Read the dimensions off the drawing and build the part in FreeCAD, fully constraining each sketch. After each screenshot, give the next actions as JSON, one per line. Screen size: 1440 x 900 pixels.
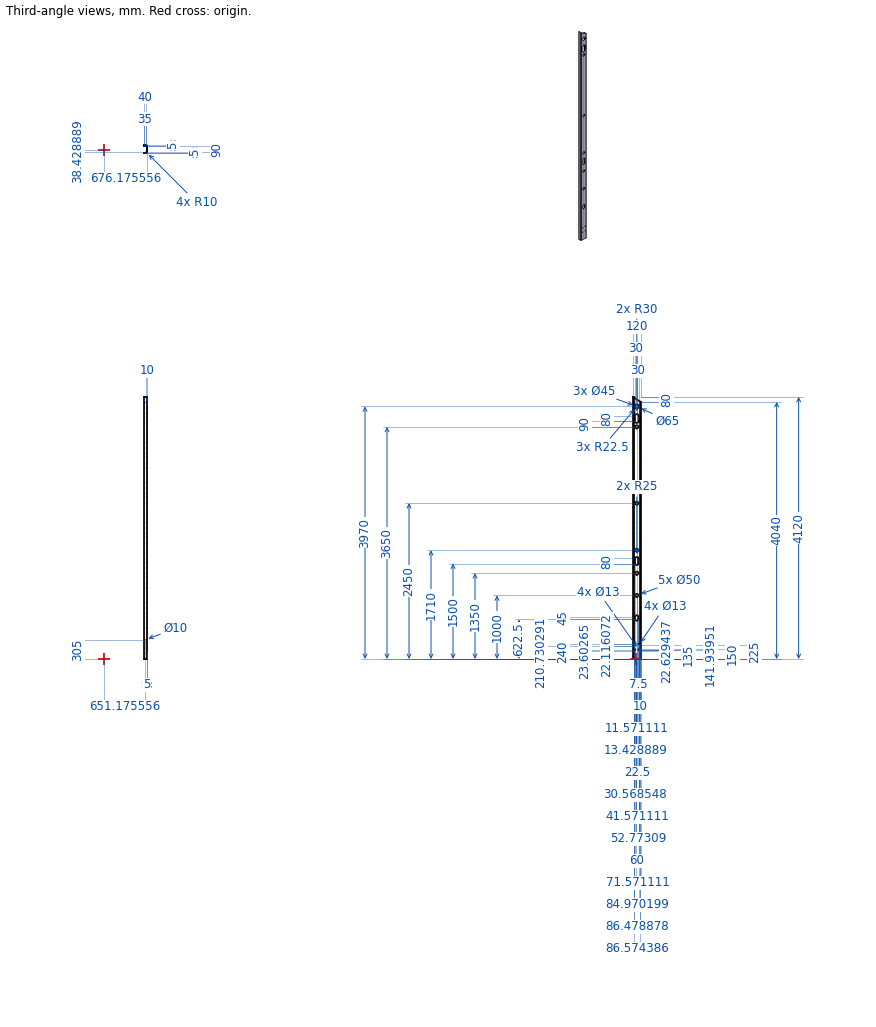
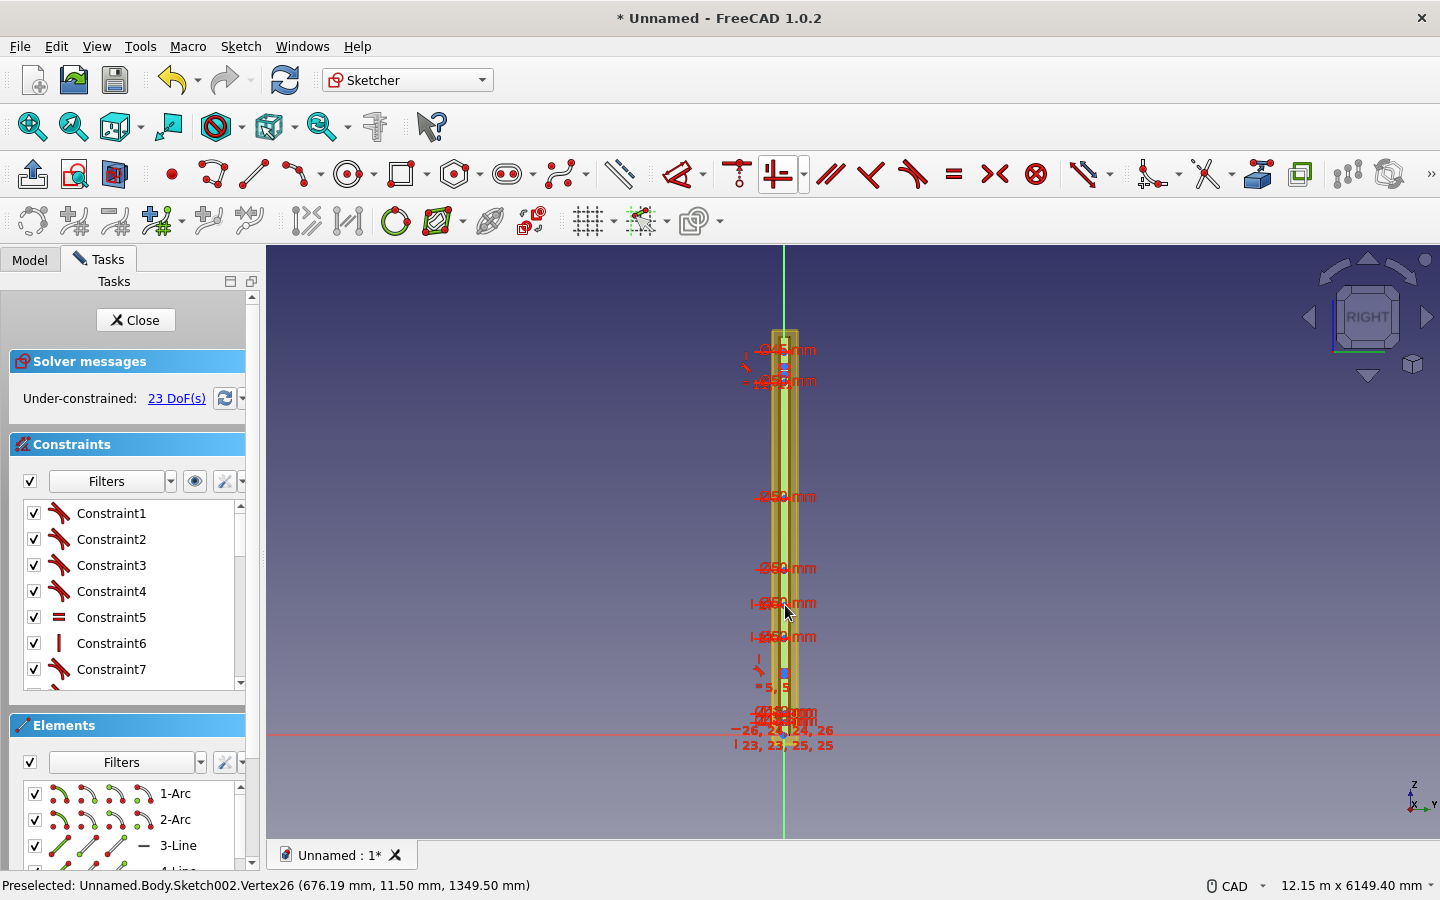
{"action": "left_click", "coordinate": [785, 605]}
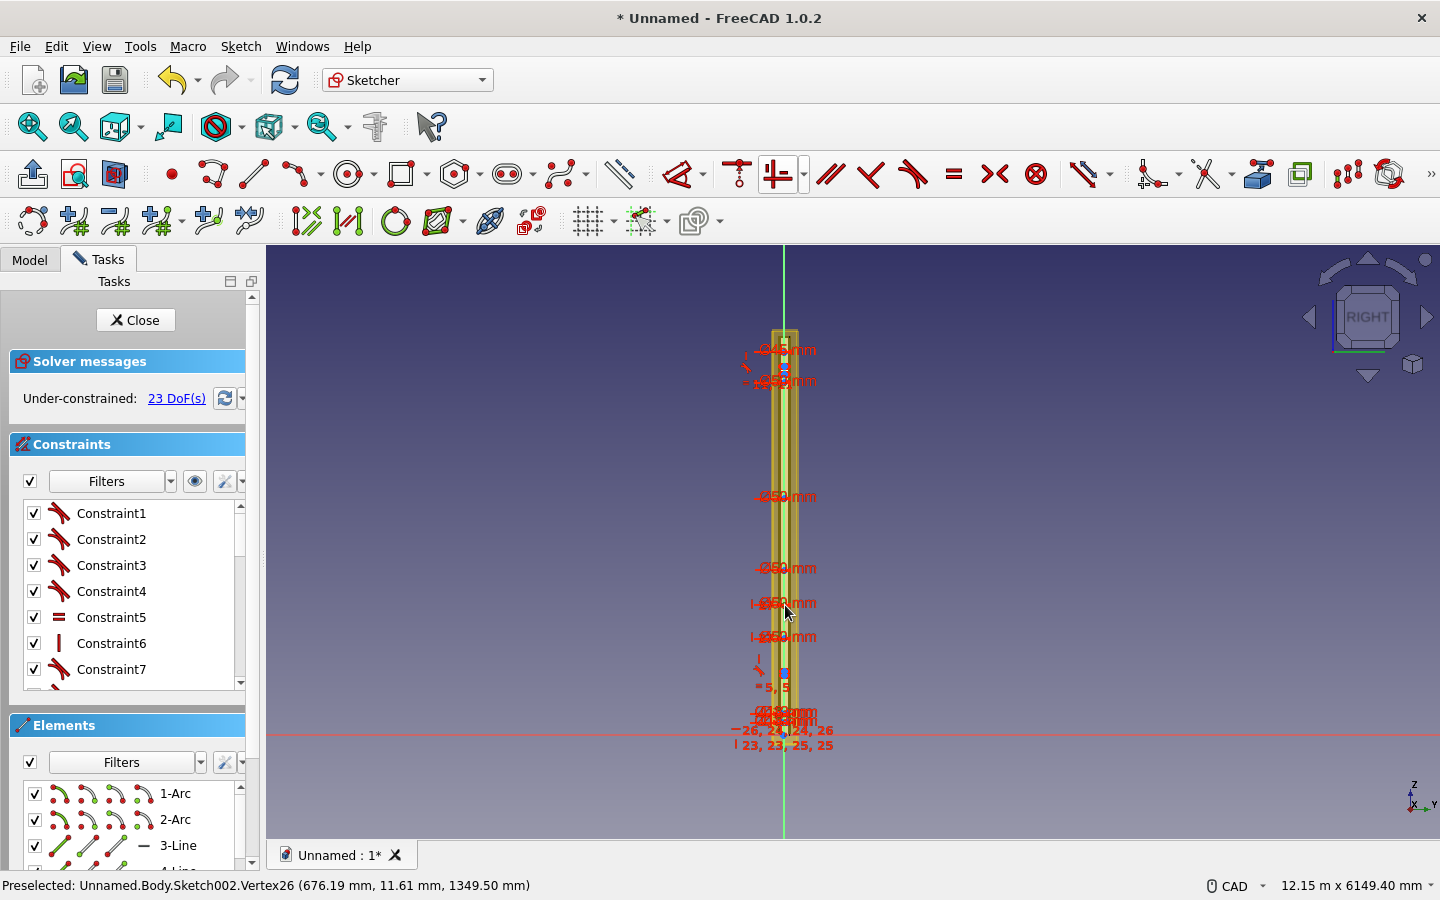
{"action": "left_click", "coordinate": [785, 570]}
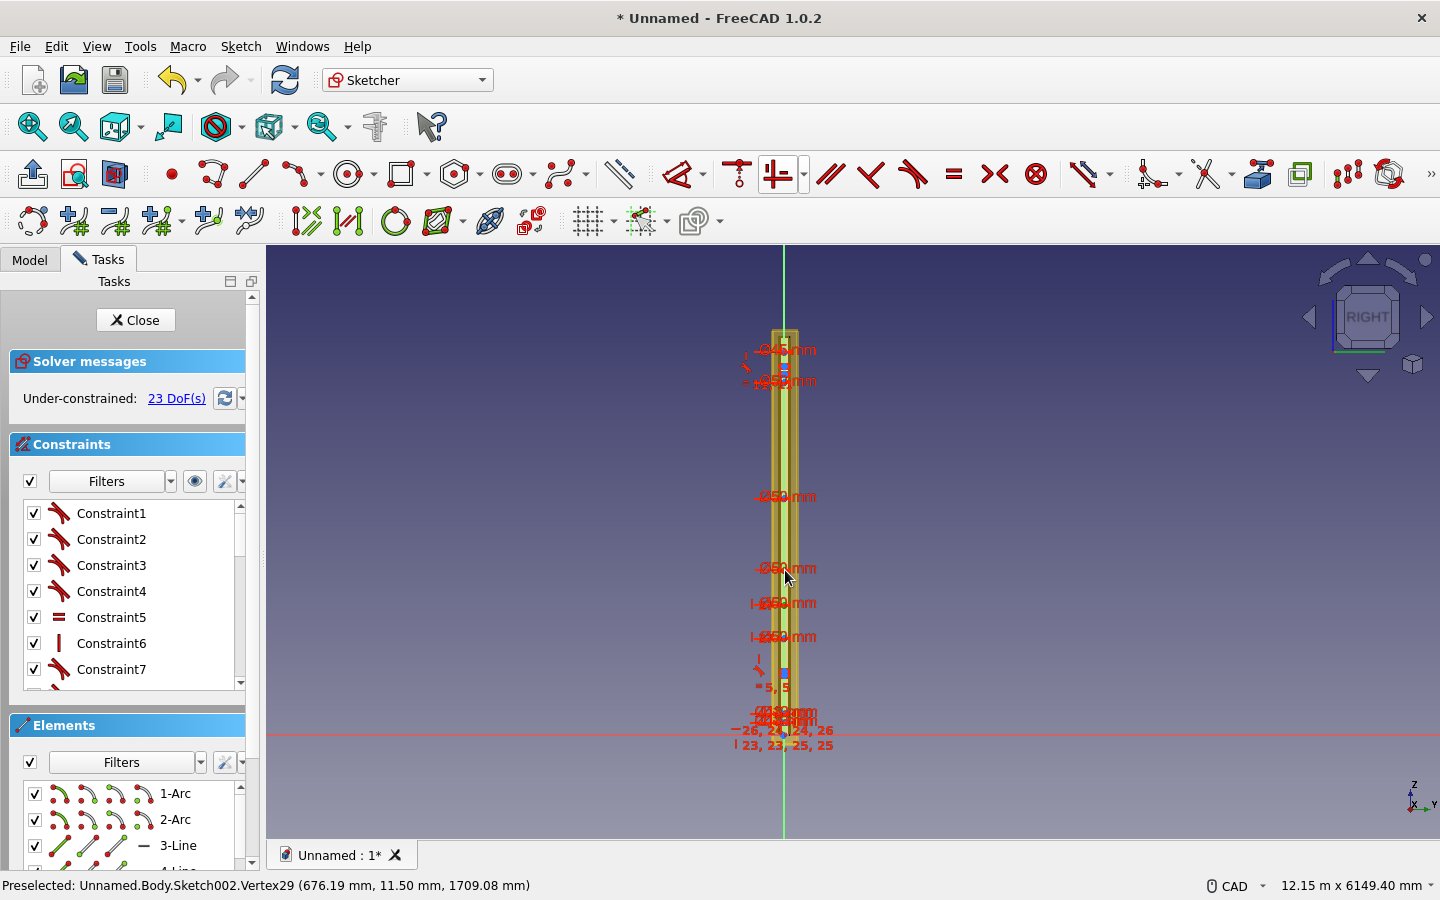
{"action": "key", "text": "v"}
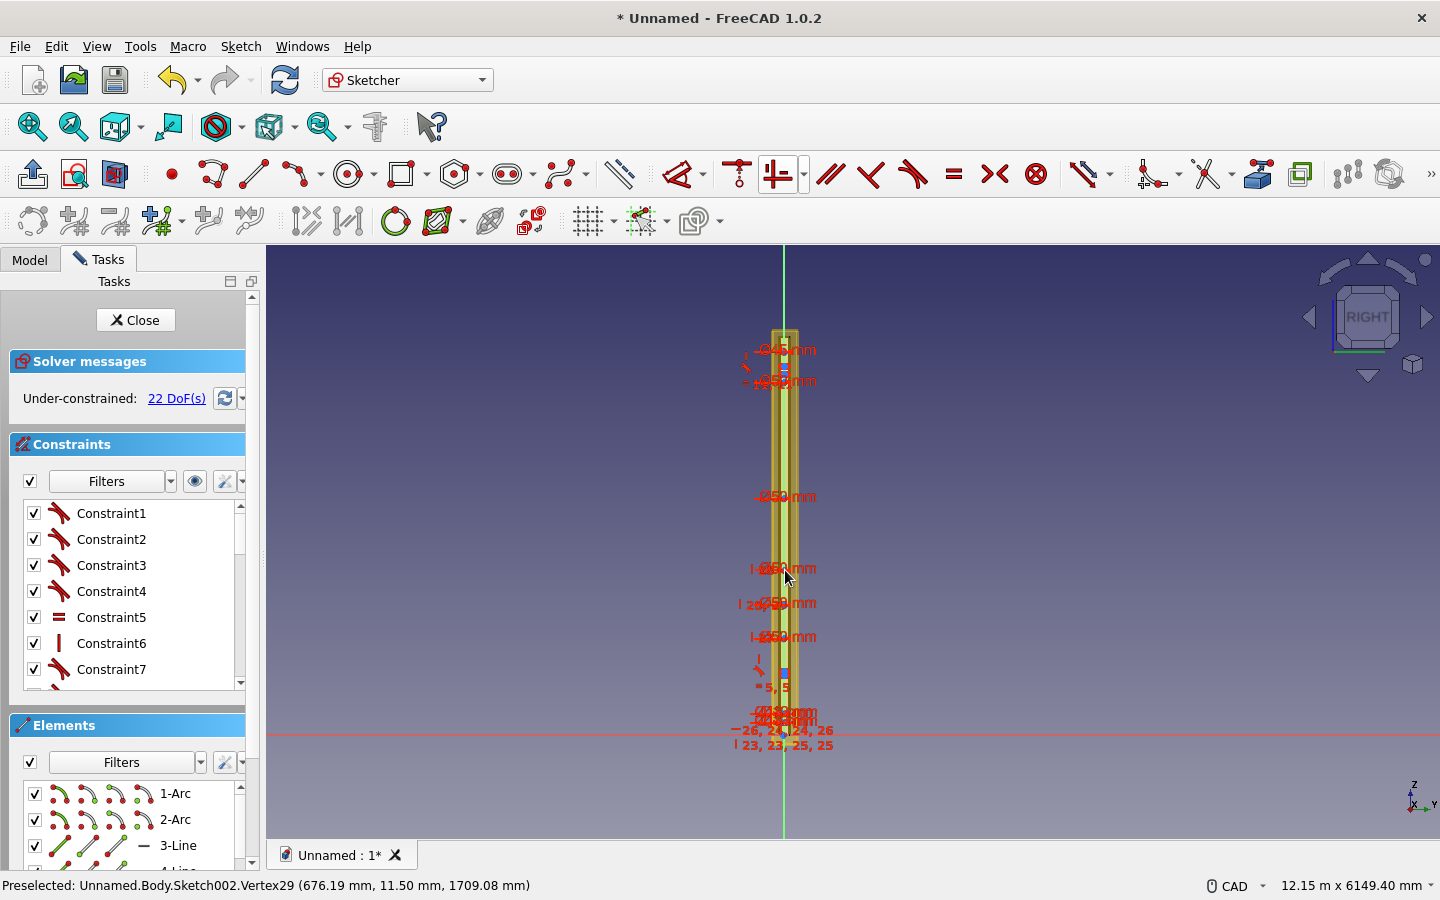
{"action": "left_click", "coordinate": [785, 570]}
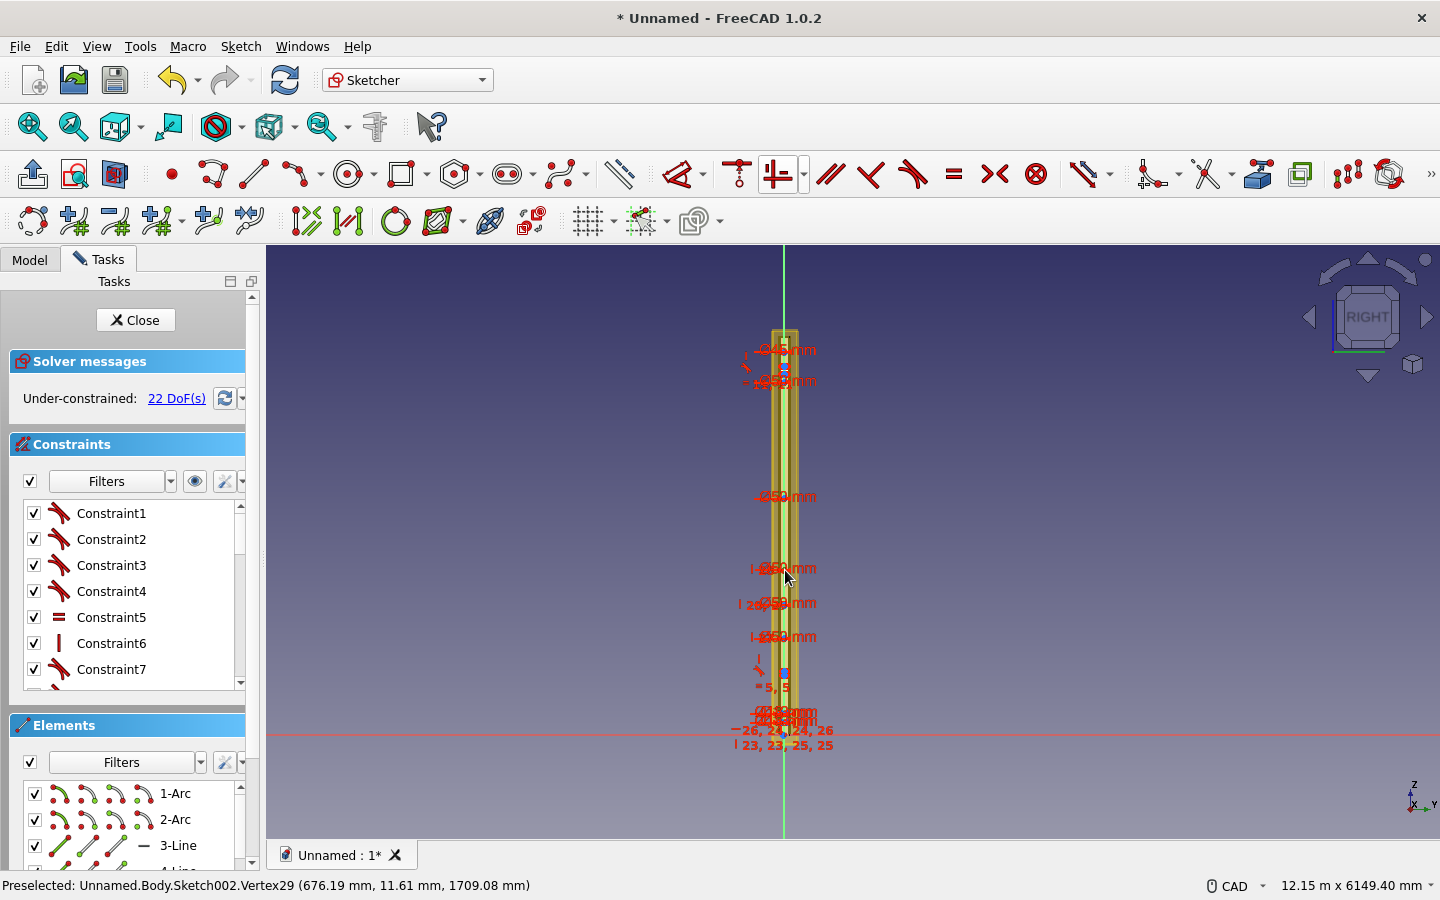
{"action": "left_click", "coordinate": [785, 499]}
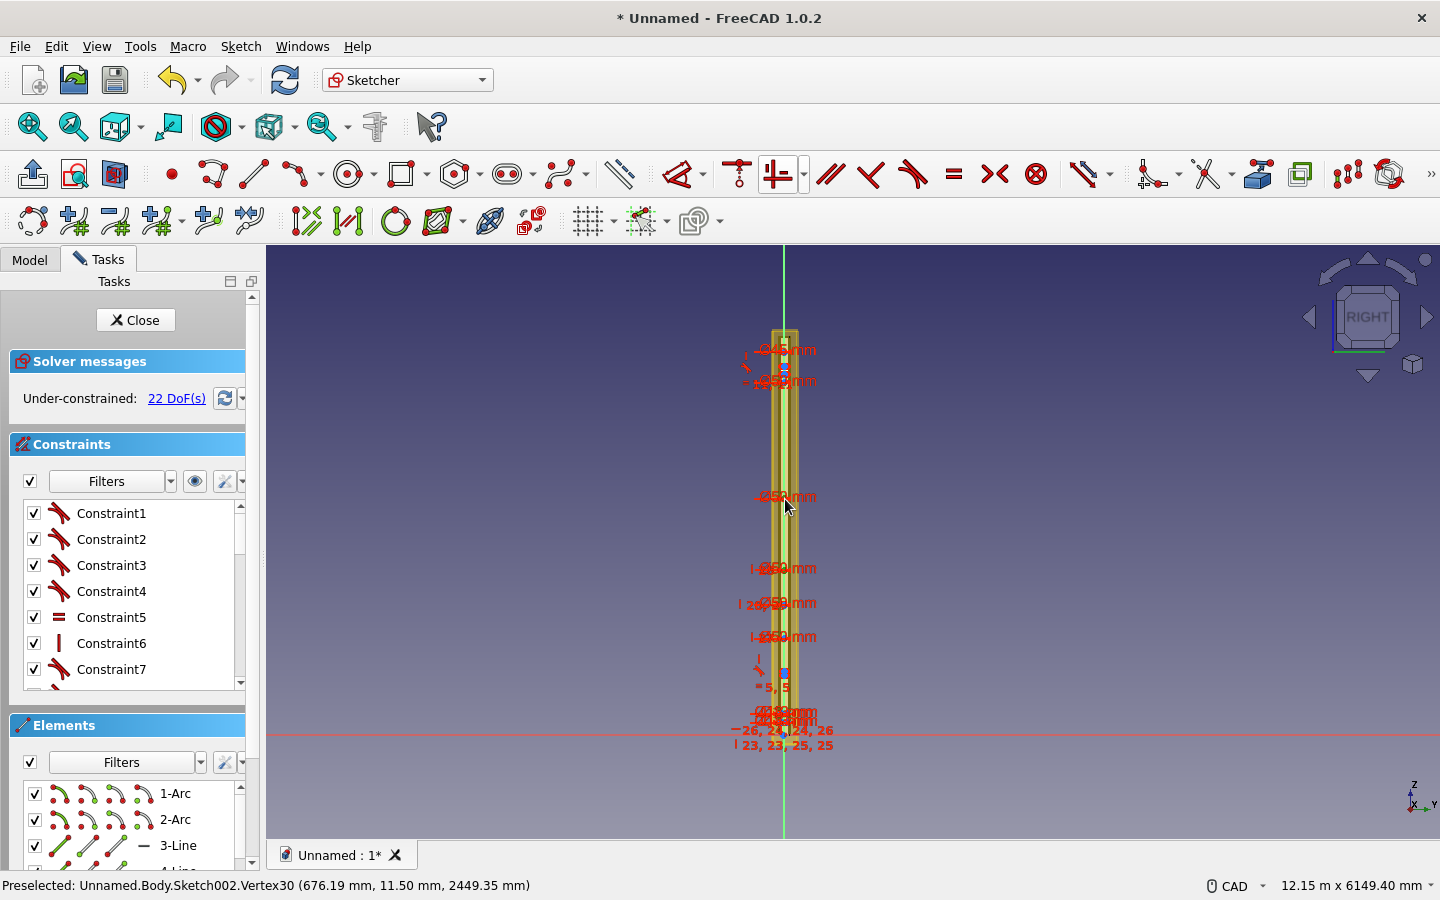
{"action": "key", "text": "v"}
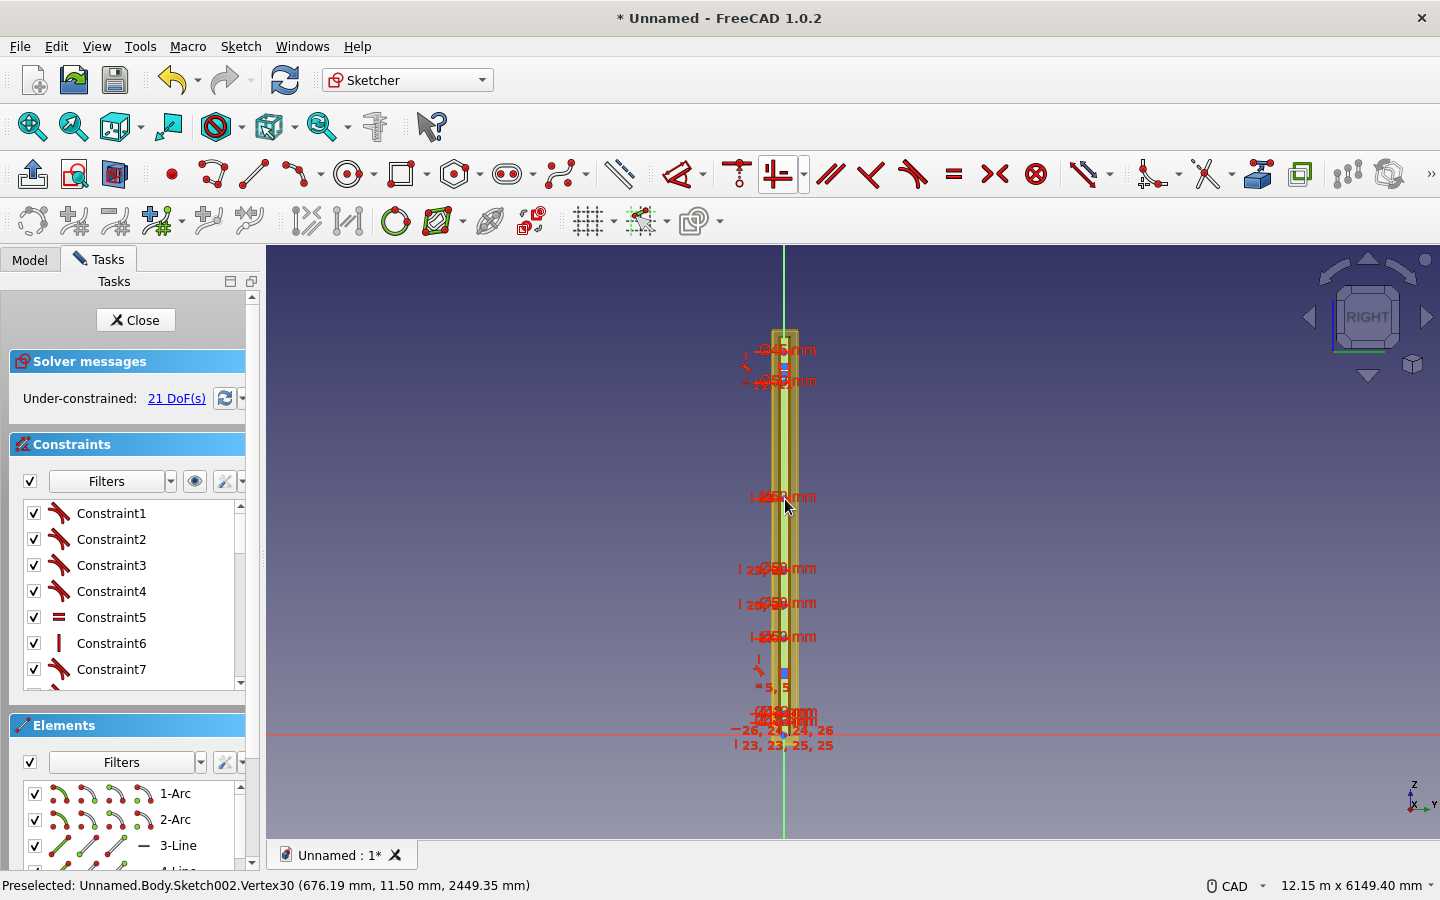
{"action": "scroll", "coordinate": [785, 383], "scroll_direction": "up", "scroll_amount": 2}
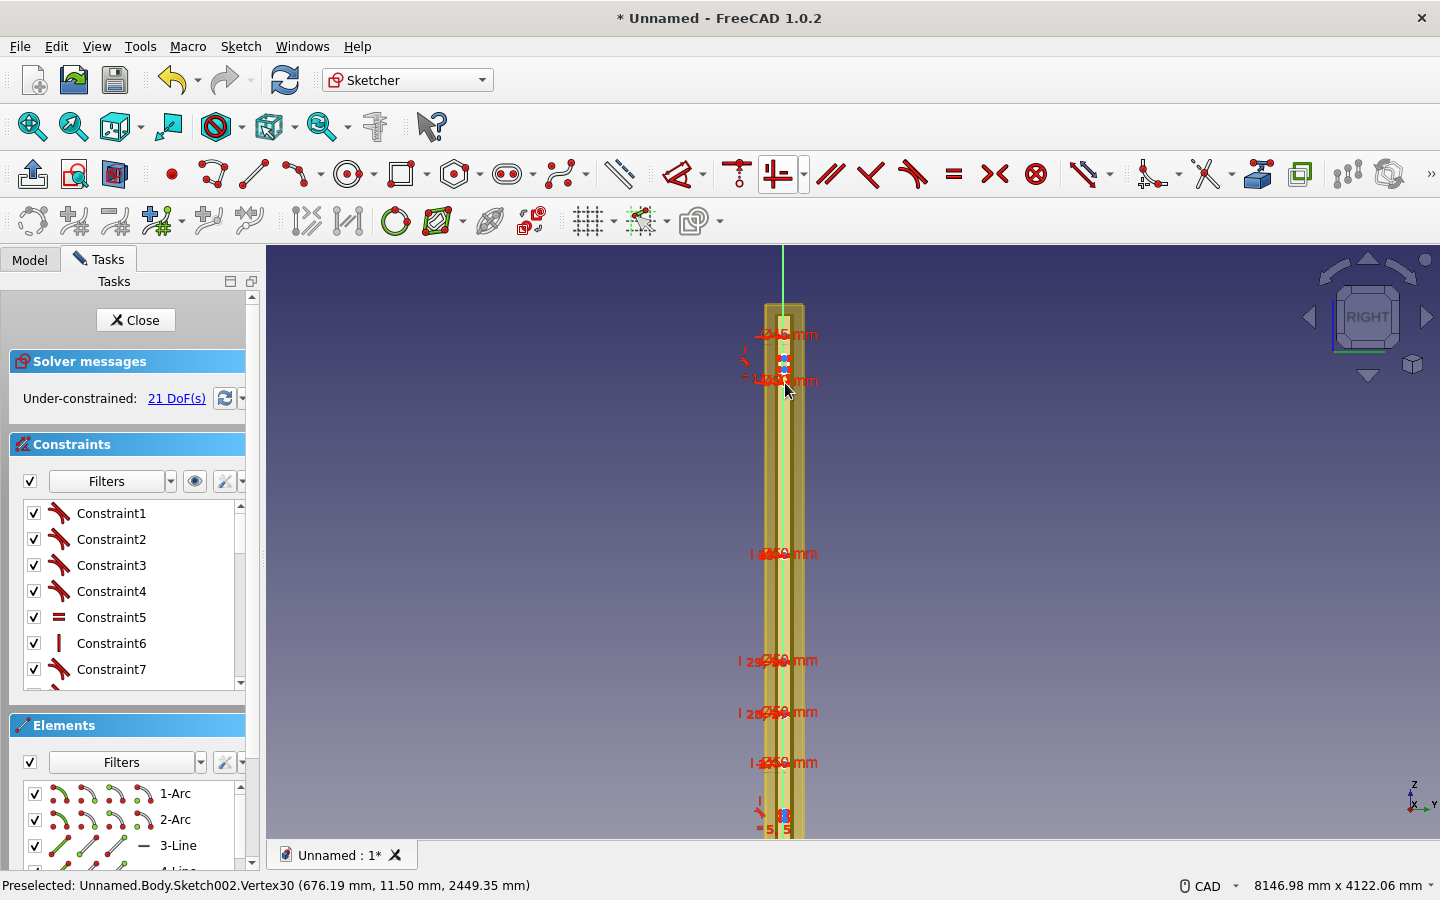
{"action": "left_click", "coordinate": [784, 383]}